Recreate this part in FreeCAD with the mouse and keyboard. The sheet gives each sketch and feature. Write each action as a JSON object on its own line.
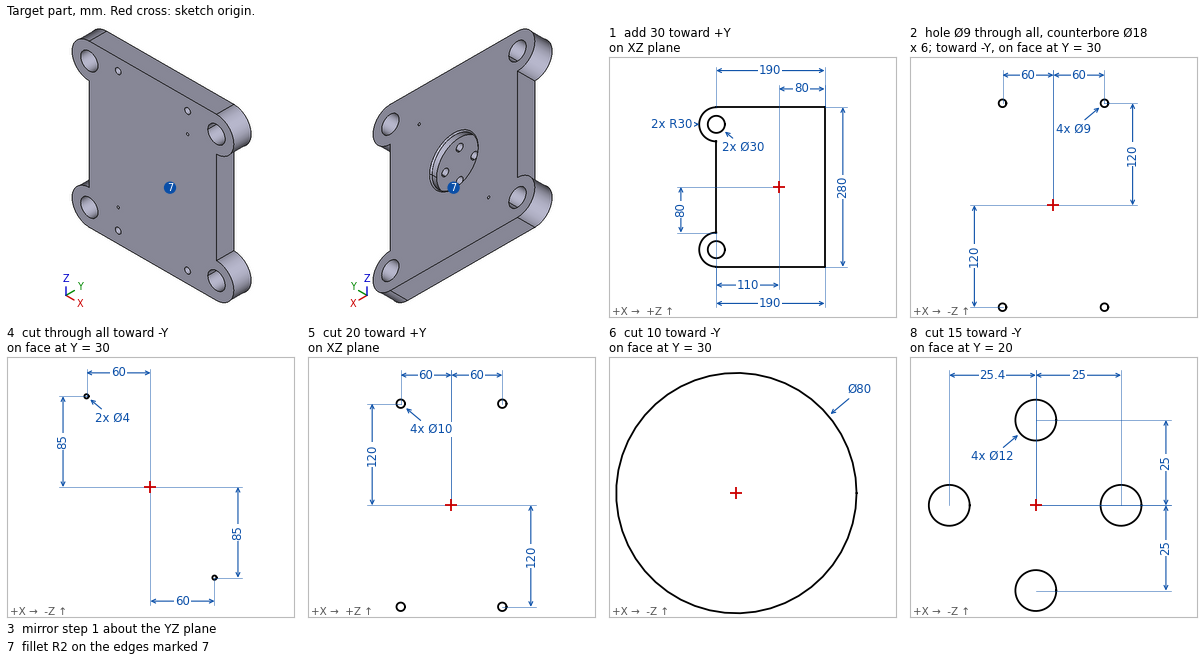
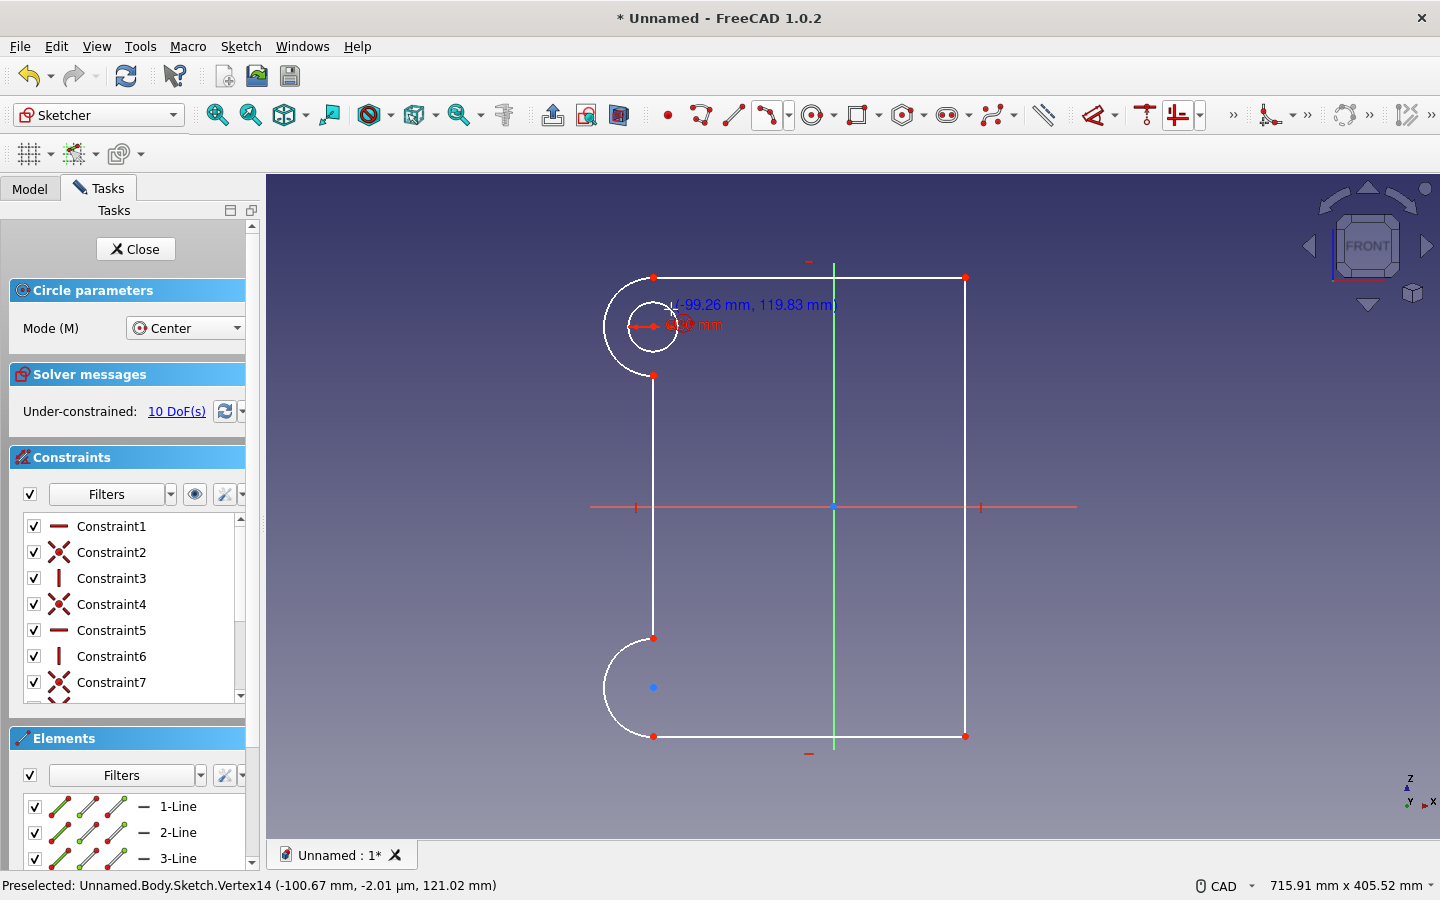
{"action": "left_click", "coordinate": [653, 687]}
{"action": "mouse_move", "coordinate": [671, 669]}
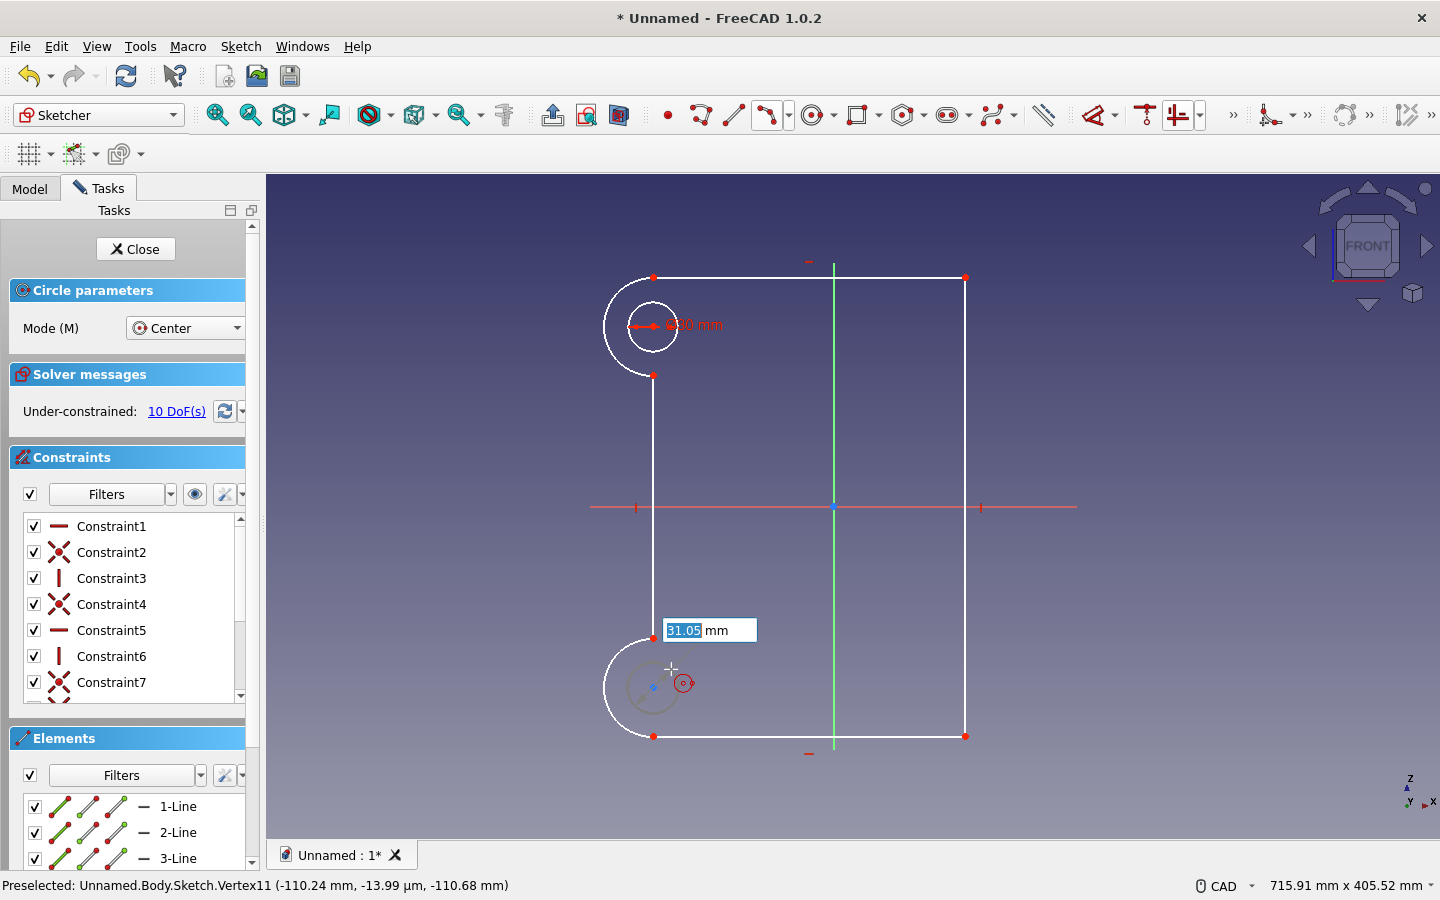
{"action": "type", "text": "30"}
{"action": "key", "text": "Return"}
{"action": "key", "text": "Escape"}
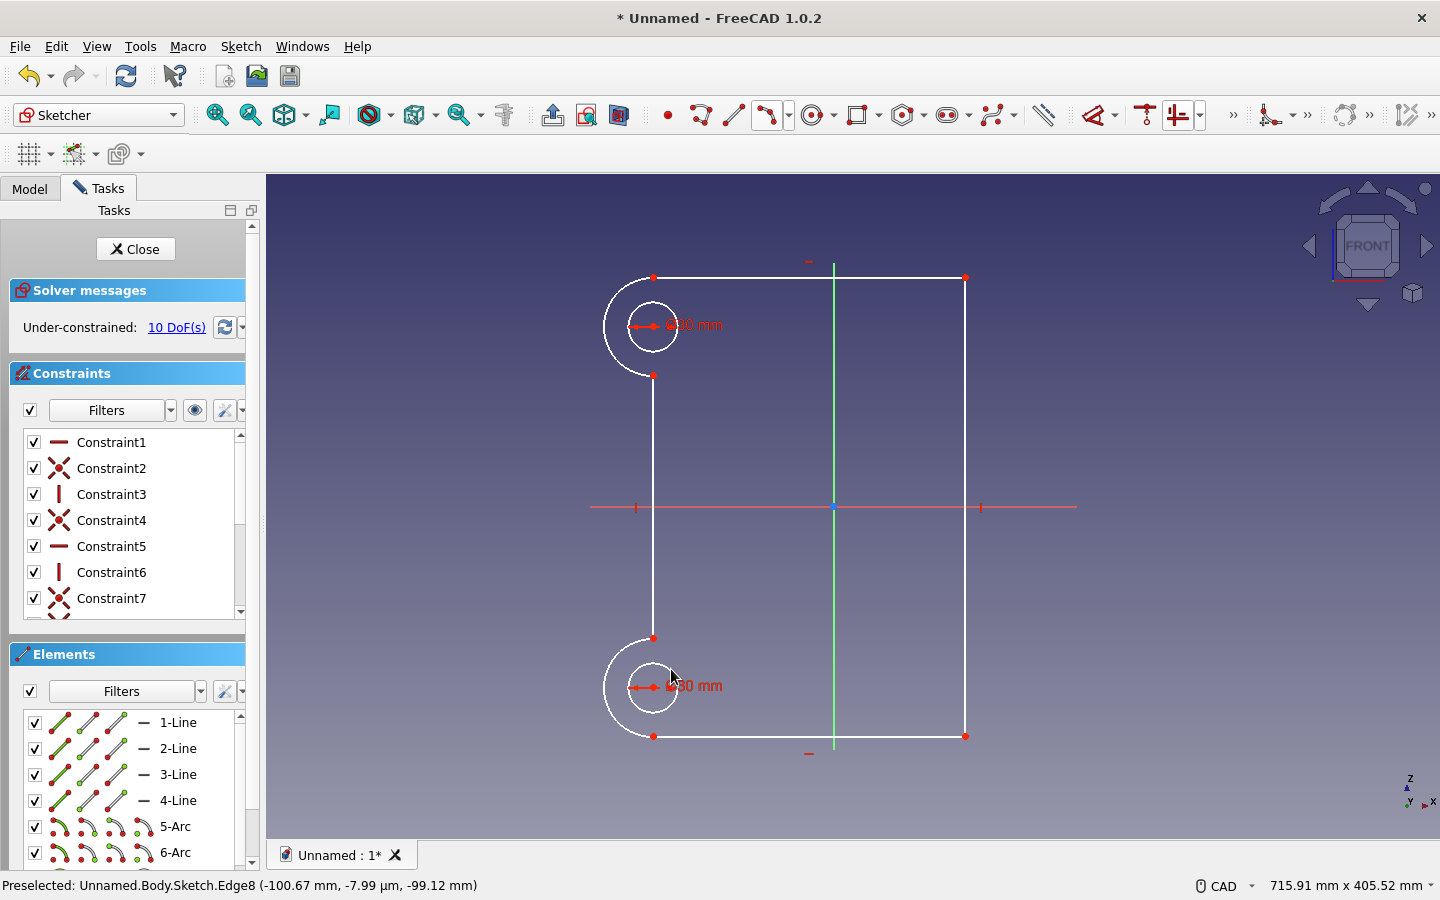
{"action": "left_click", "coordinate": [747, 278]}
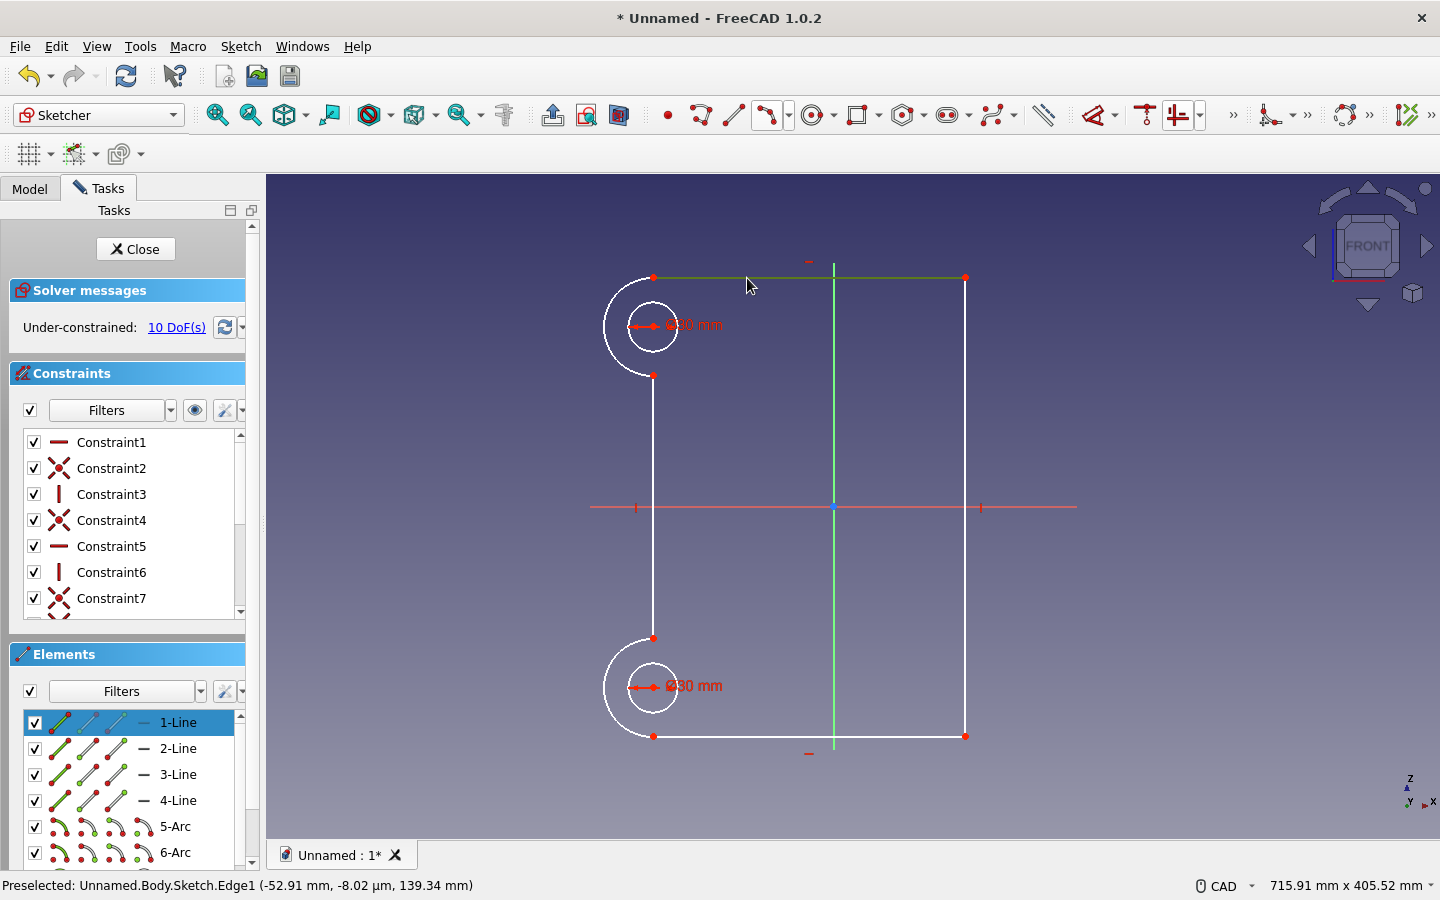
{"action": "left_click", "coordinate": [613, 298]}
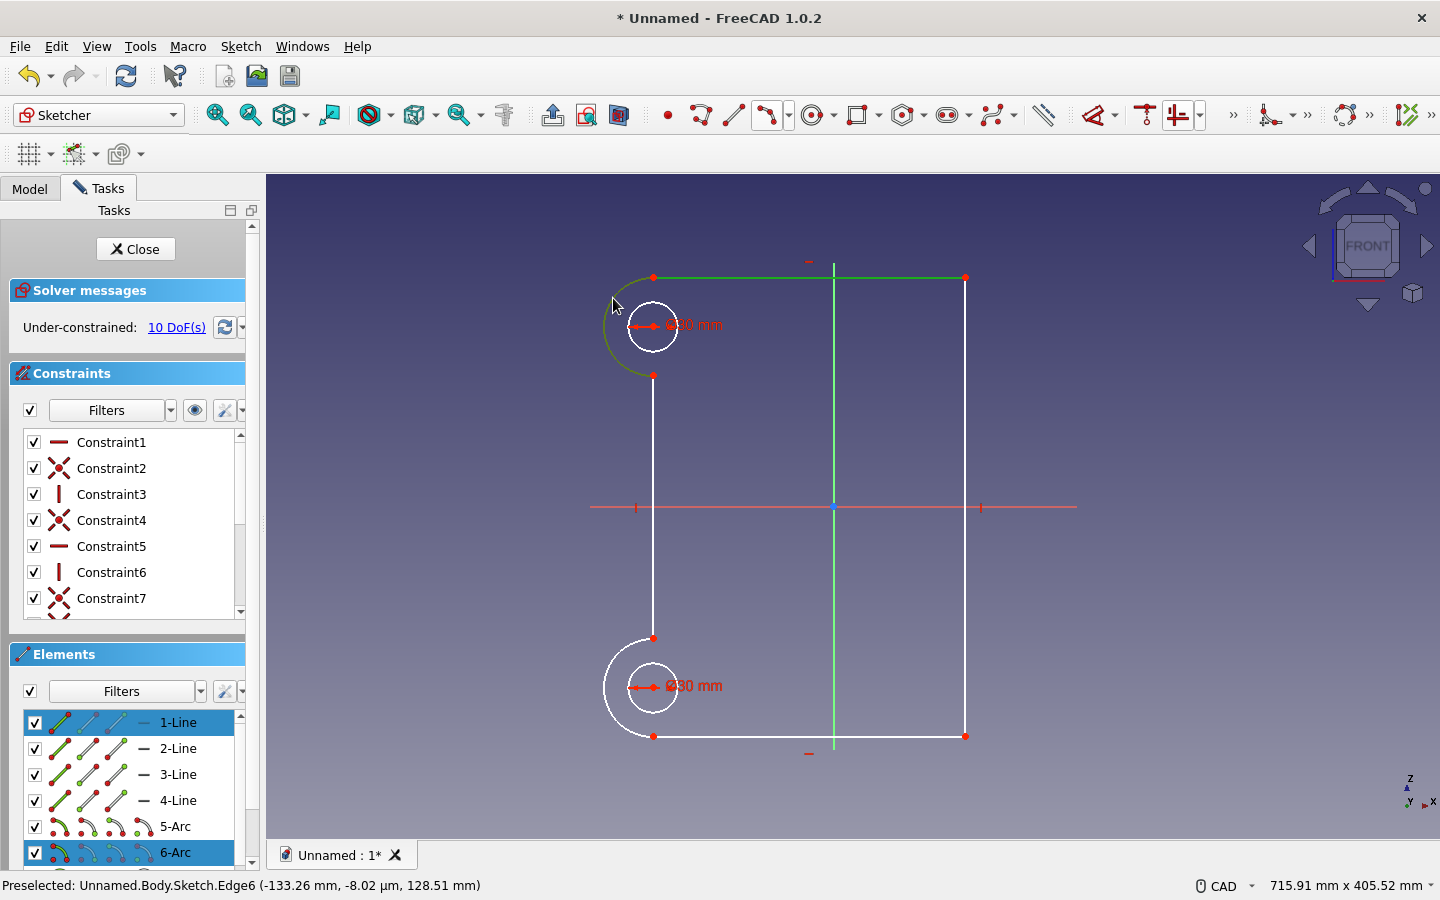
{"action": "key", "text": "t"}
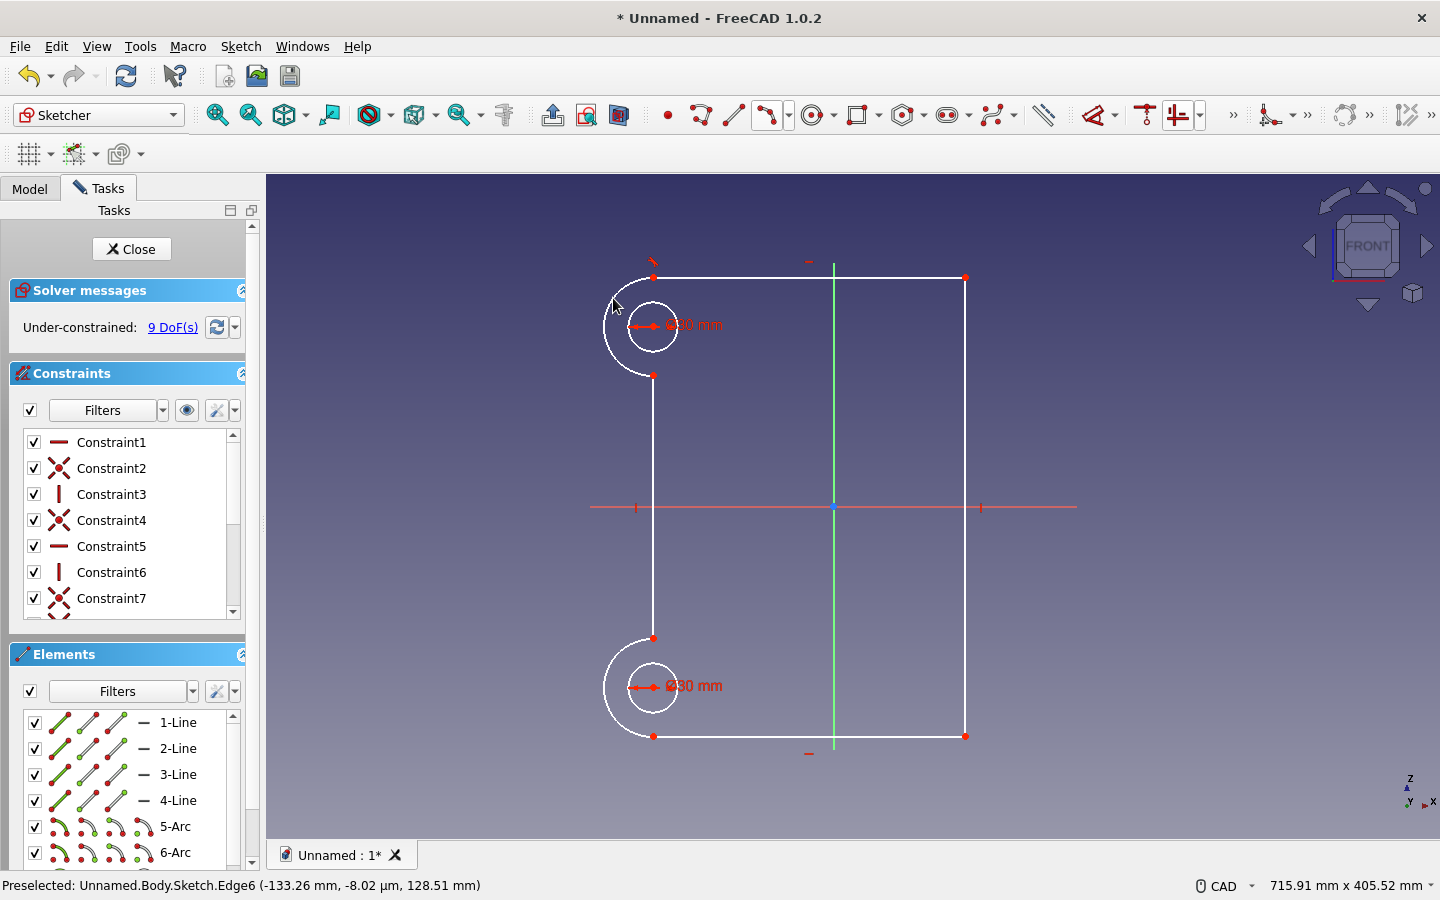
{"action": "left_click", "coordinate": [871, 737]}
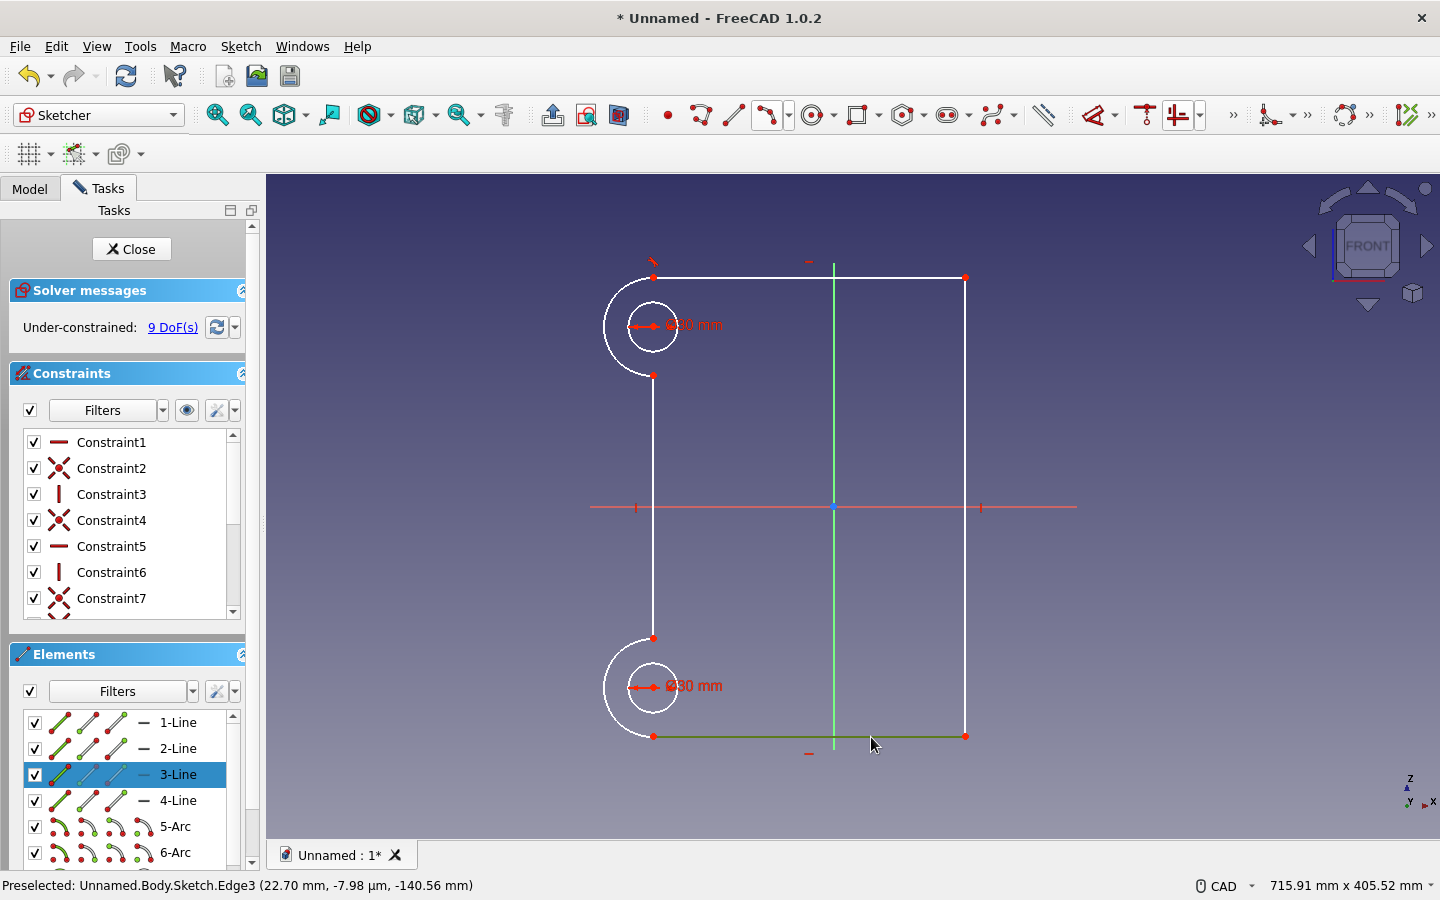
{"action": "left_click", "coordinate": [613, 659]}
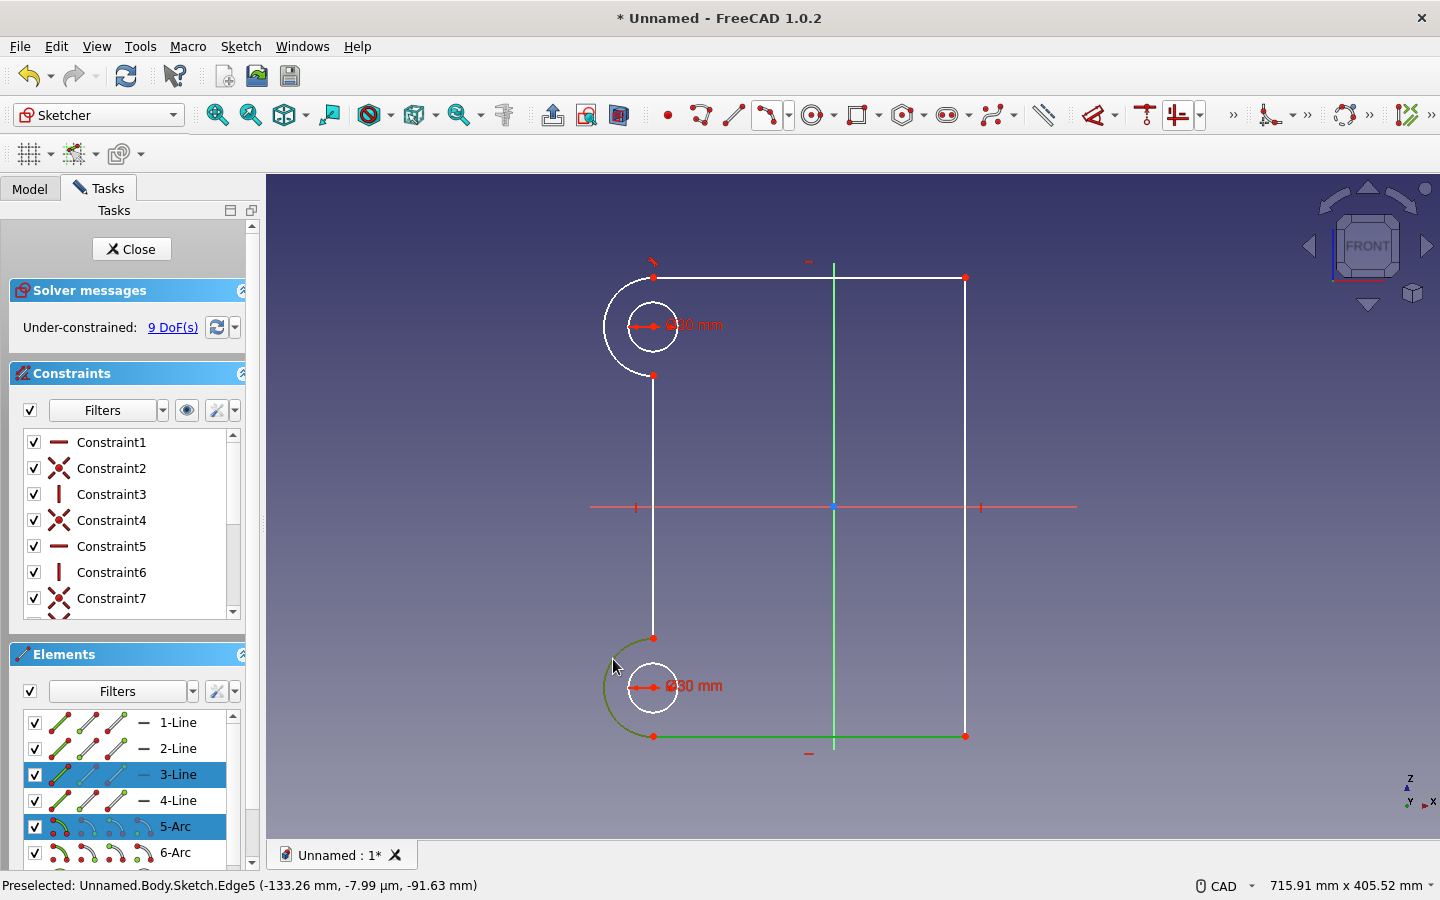
{"action": "key", "text": "t"}